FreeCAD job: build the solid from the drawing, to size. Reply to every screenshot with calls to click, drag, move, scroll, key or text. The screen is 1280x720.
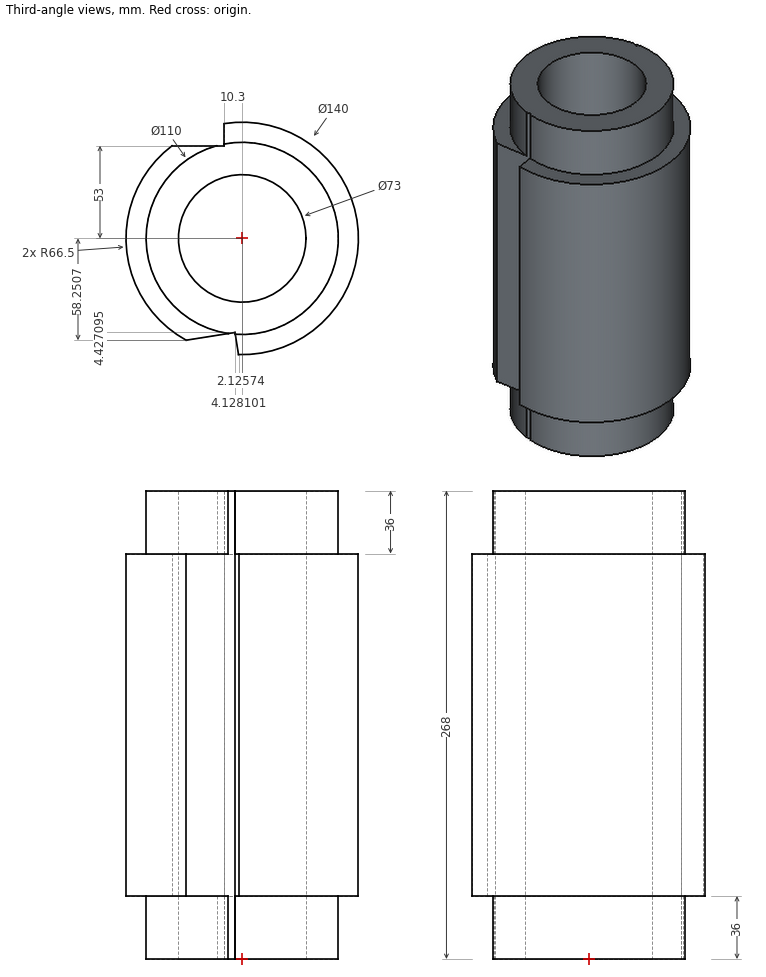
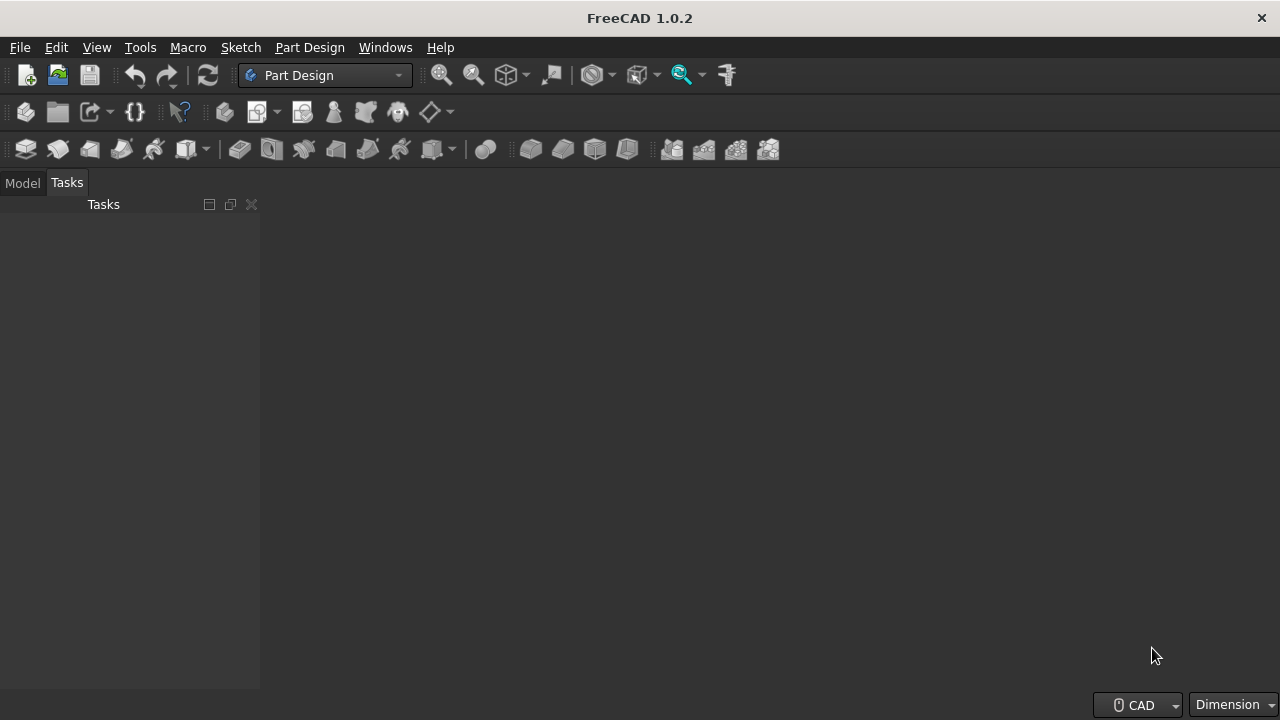
click(26, 76)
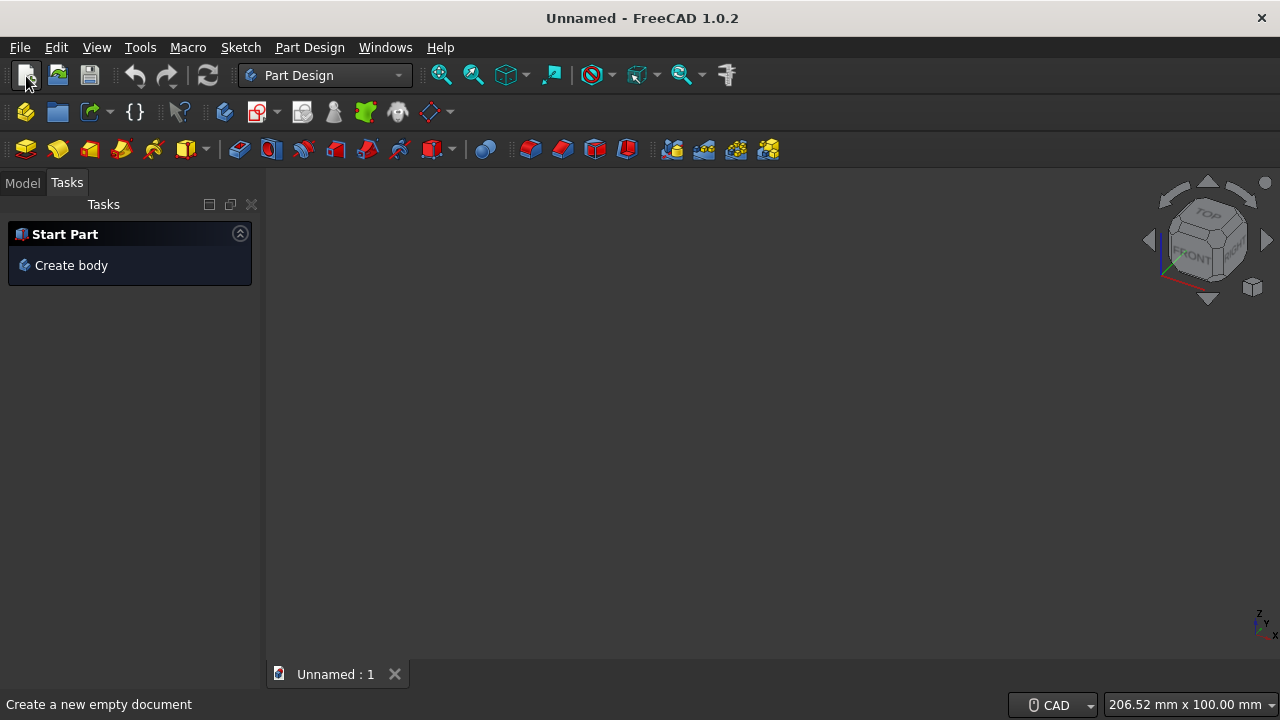
click(258, 112)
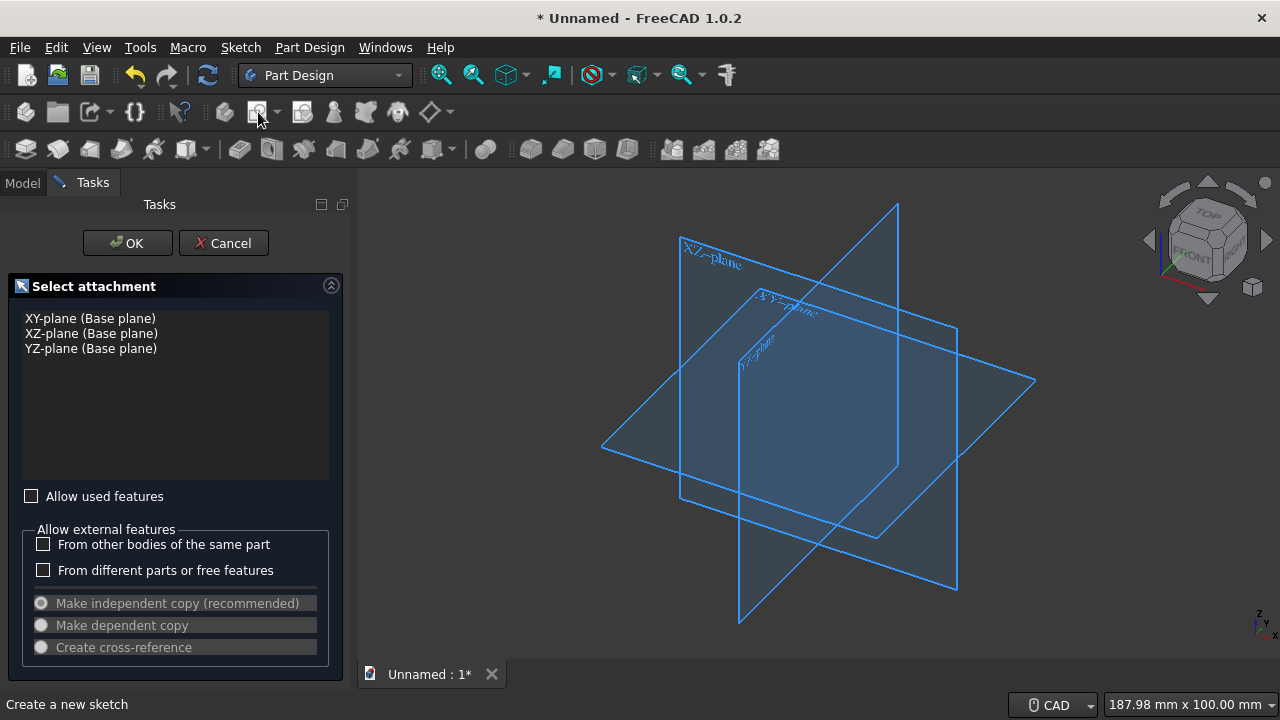
click(82, 318)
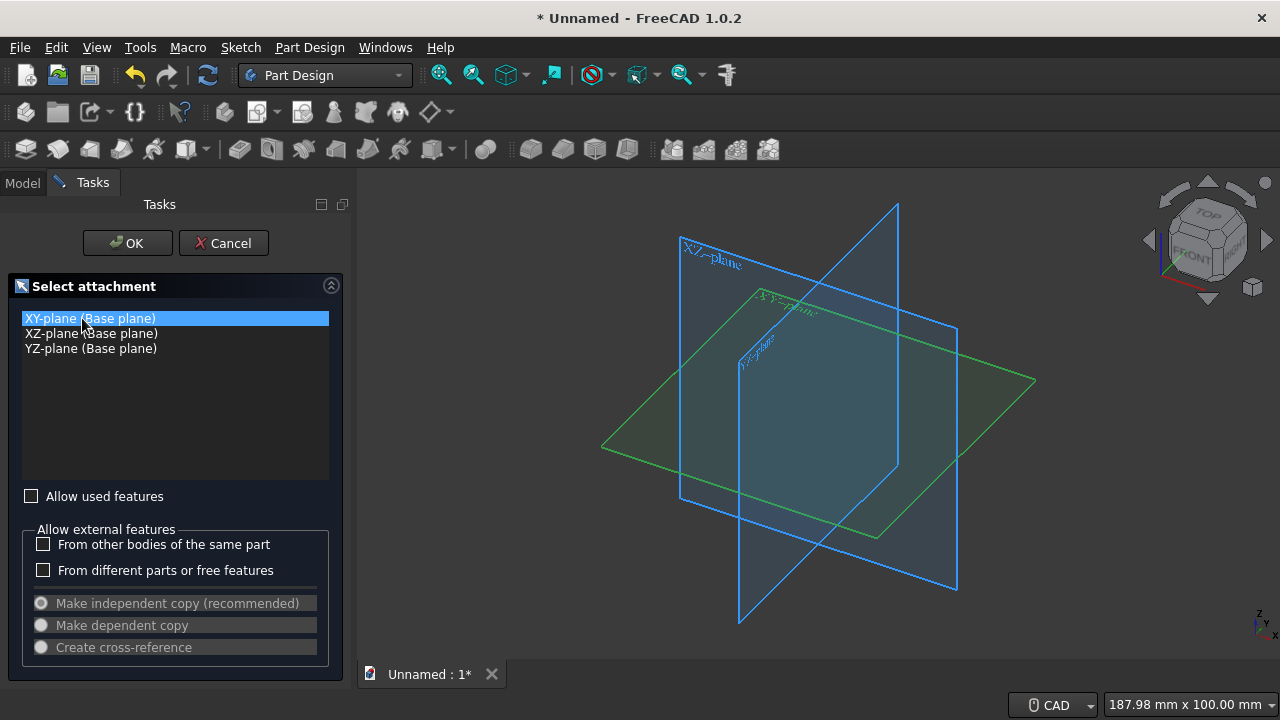
click(128, 243)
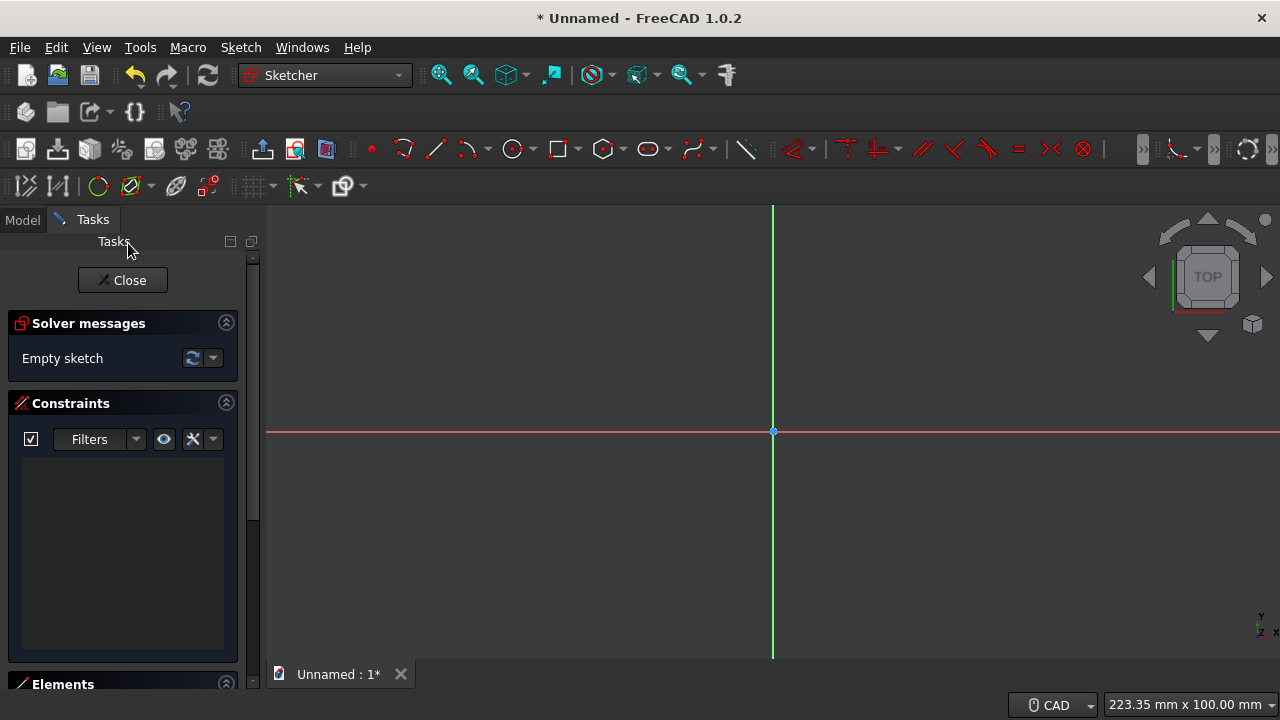
scroll(649, 431, down, 4)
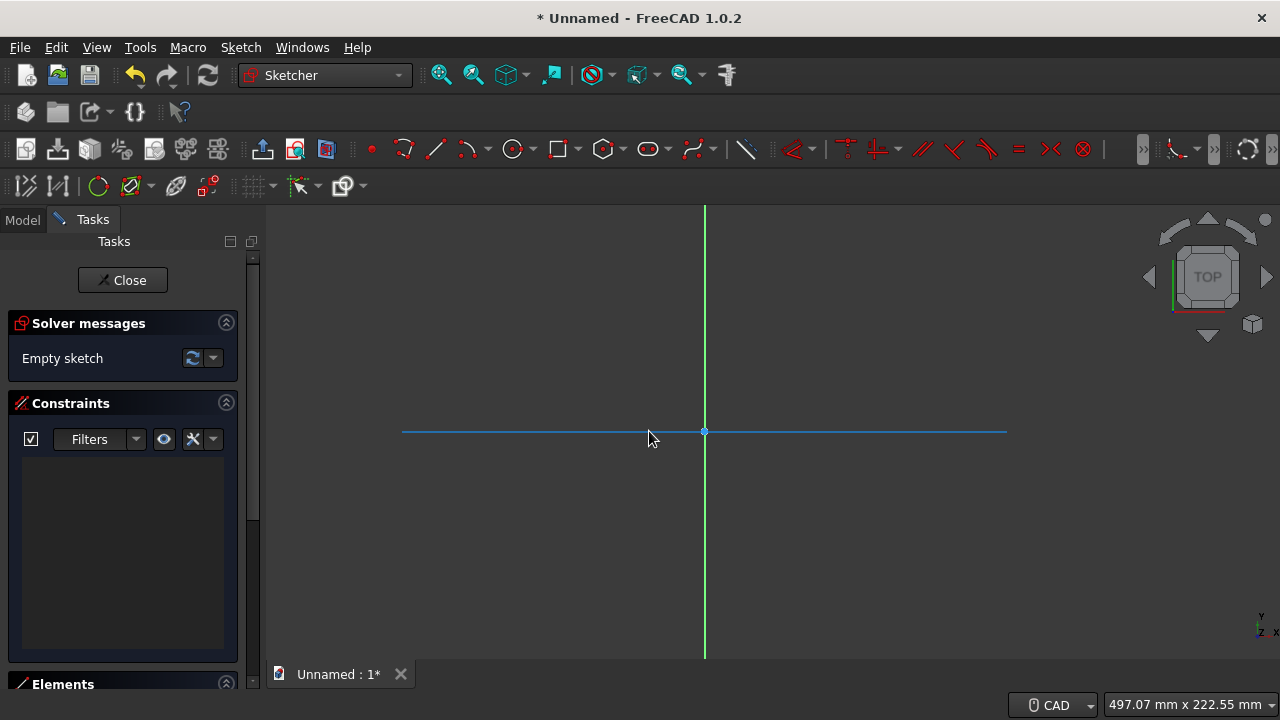
click(404, 150)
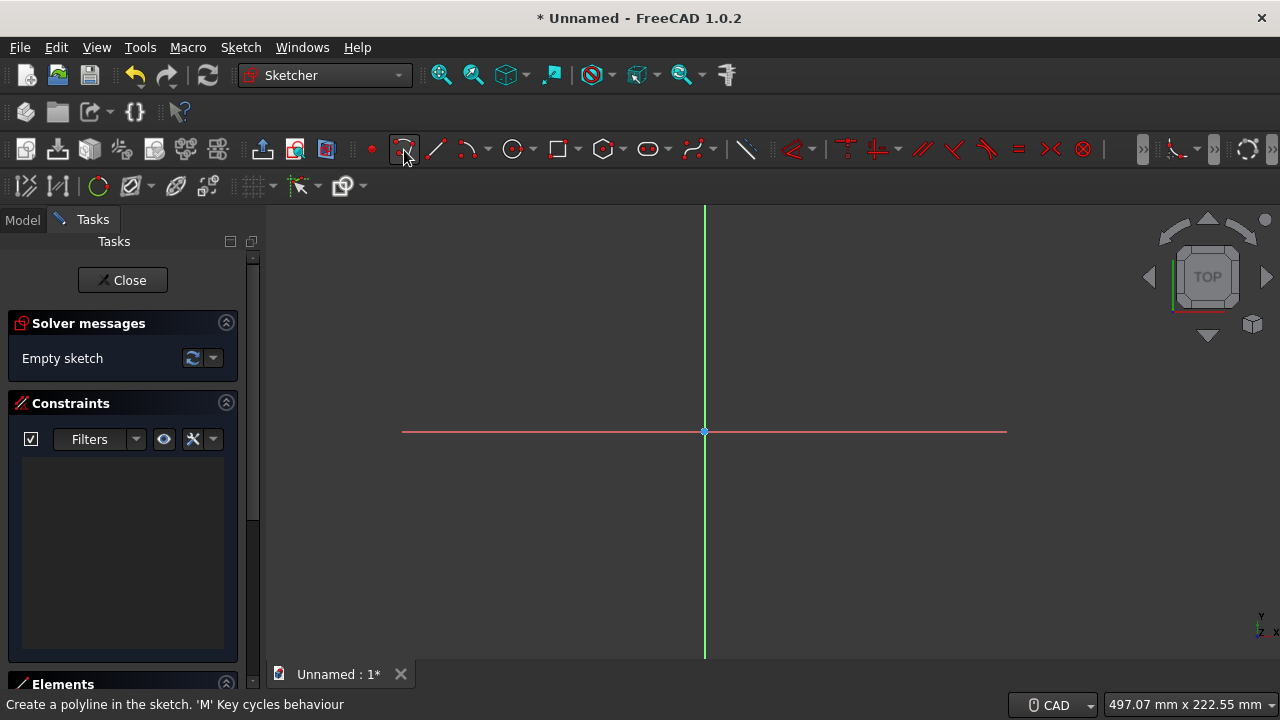
click(639, 551)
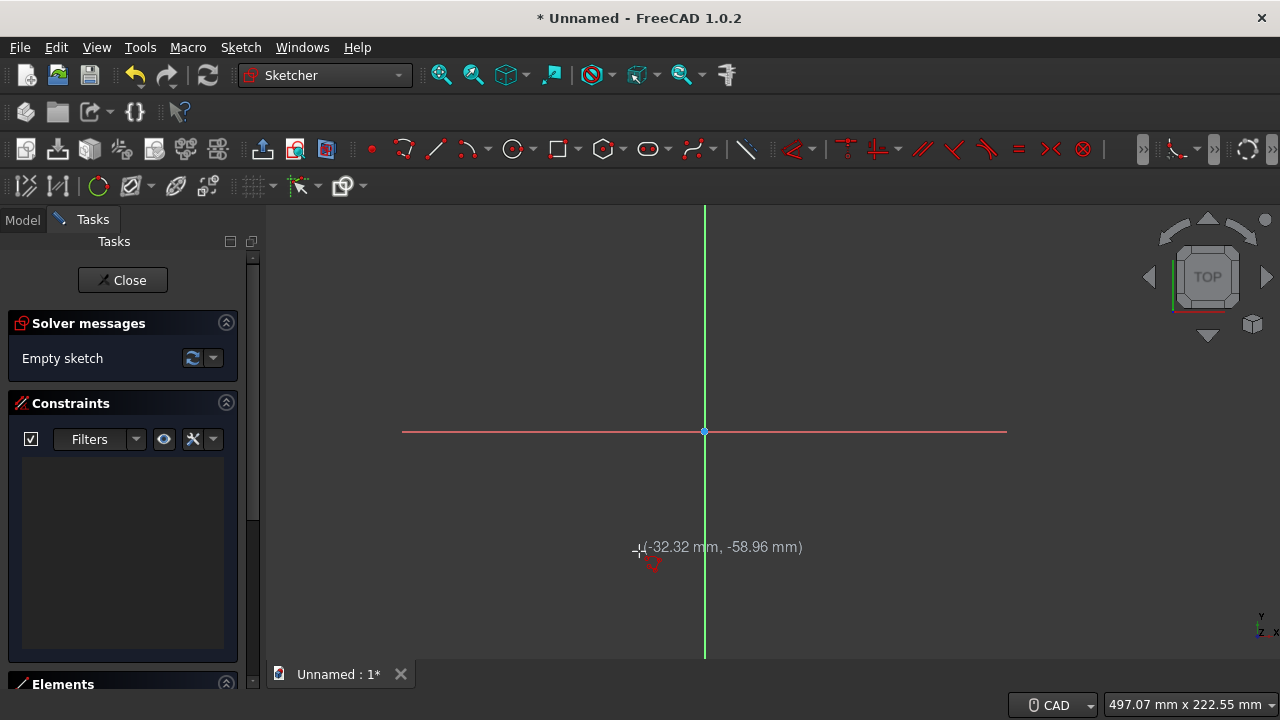
scroll(697, 542, up, 4)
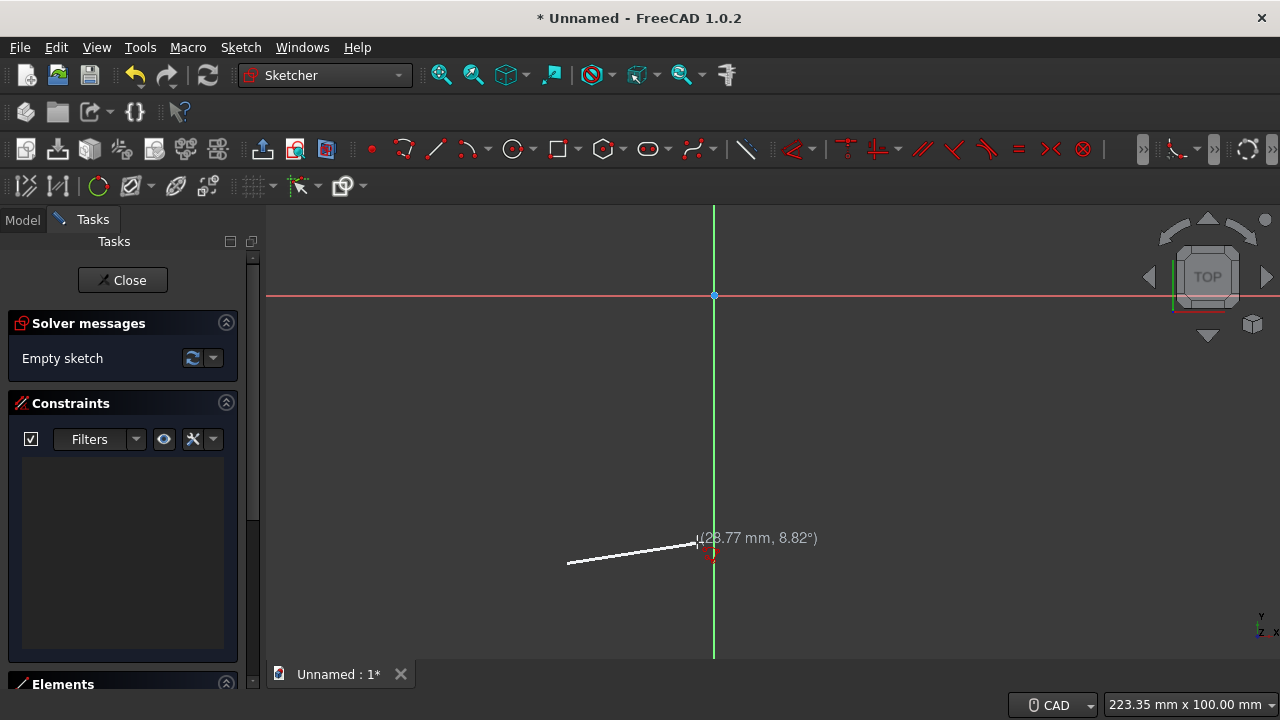
click(695, 540)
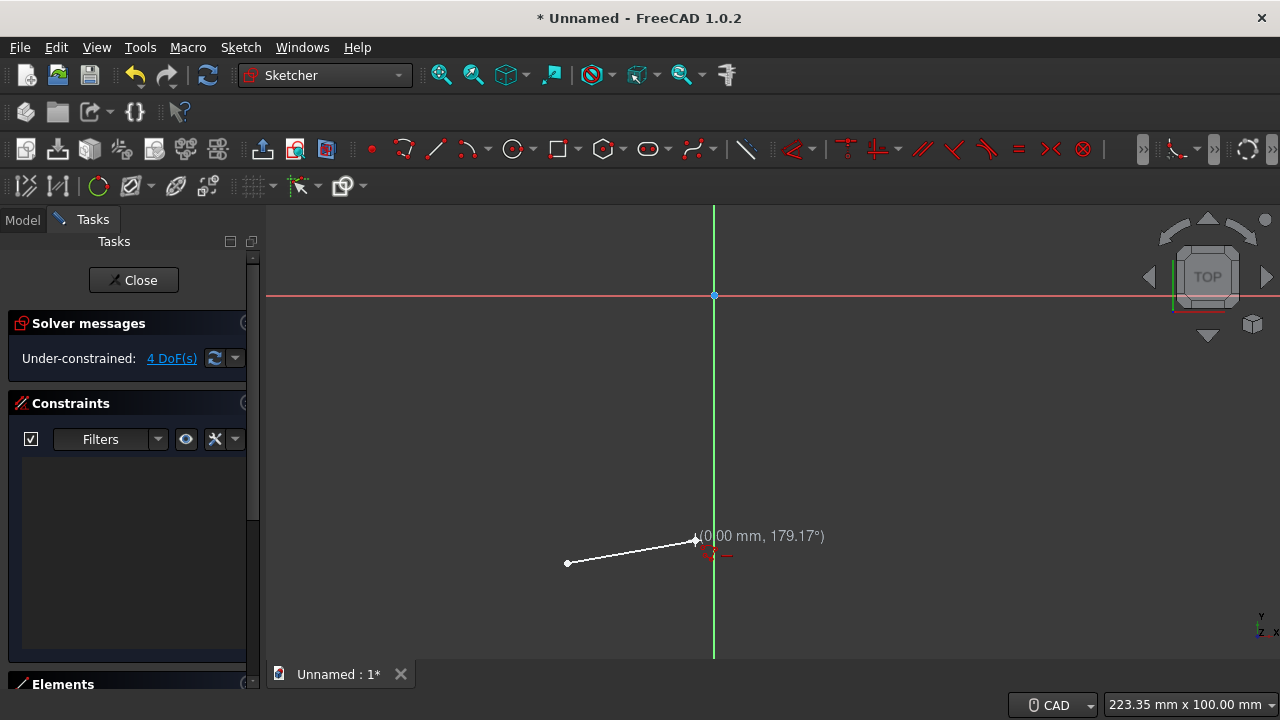
scroll(704, 597, up, 3)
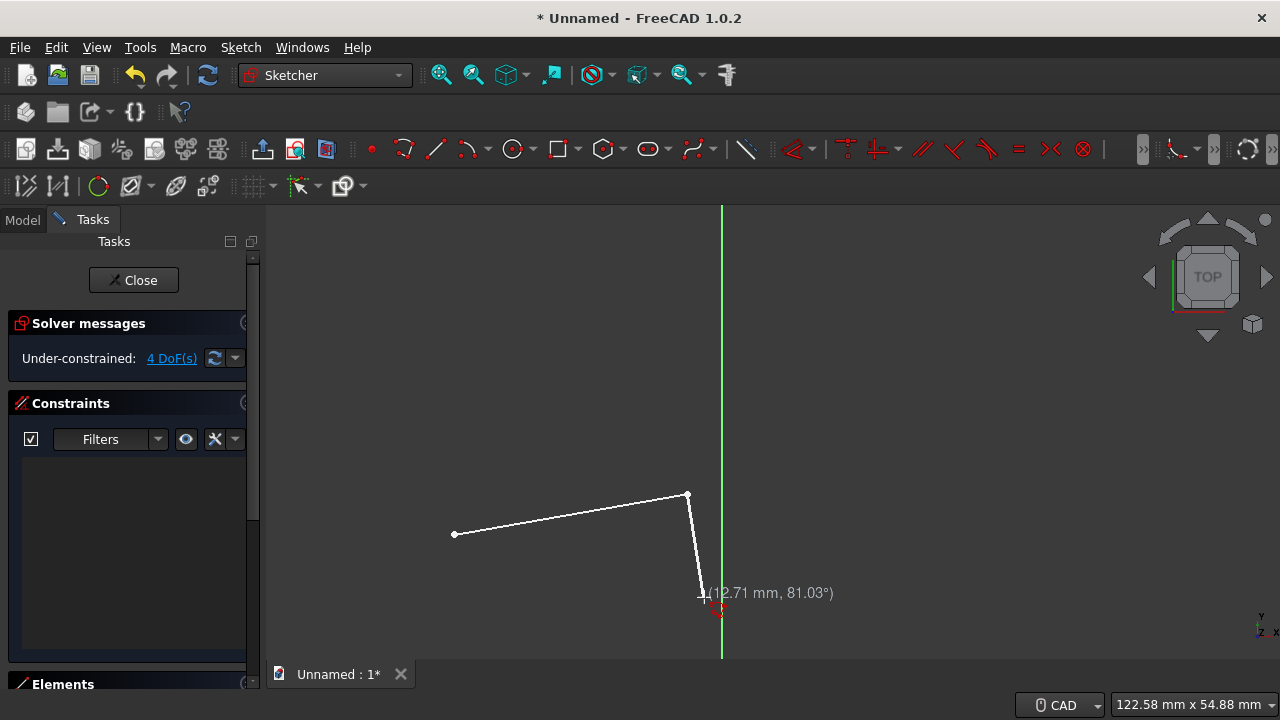
click(704, 597)
right_click(704, 597)